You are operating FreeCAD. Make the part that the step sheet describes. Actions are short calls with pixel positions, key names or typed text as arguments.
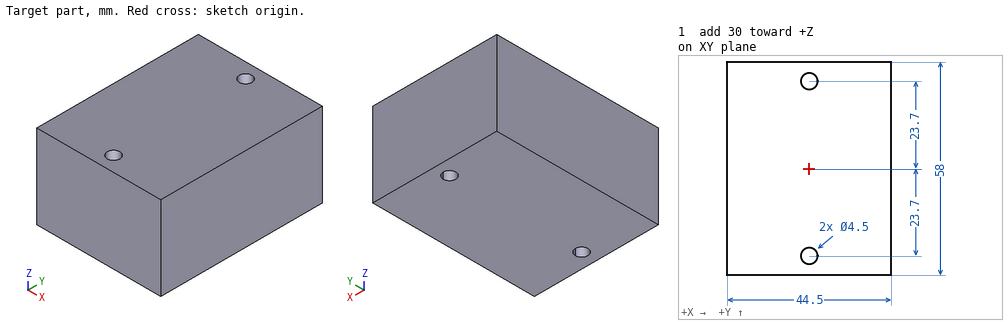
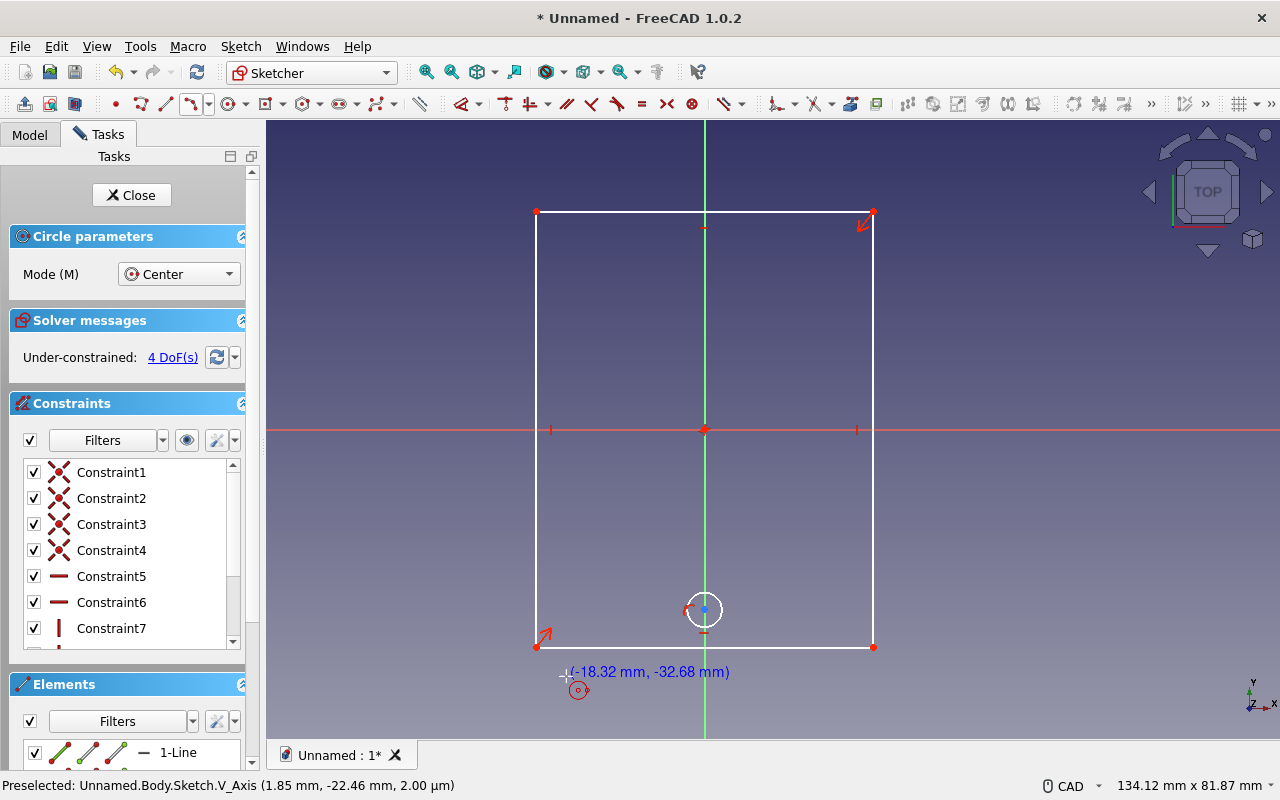
scroll(705, 251, up, 2)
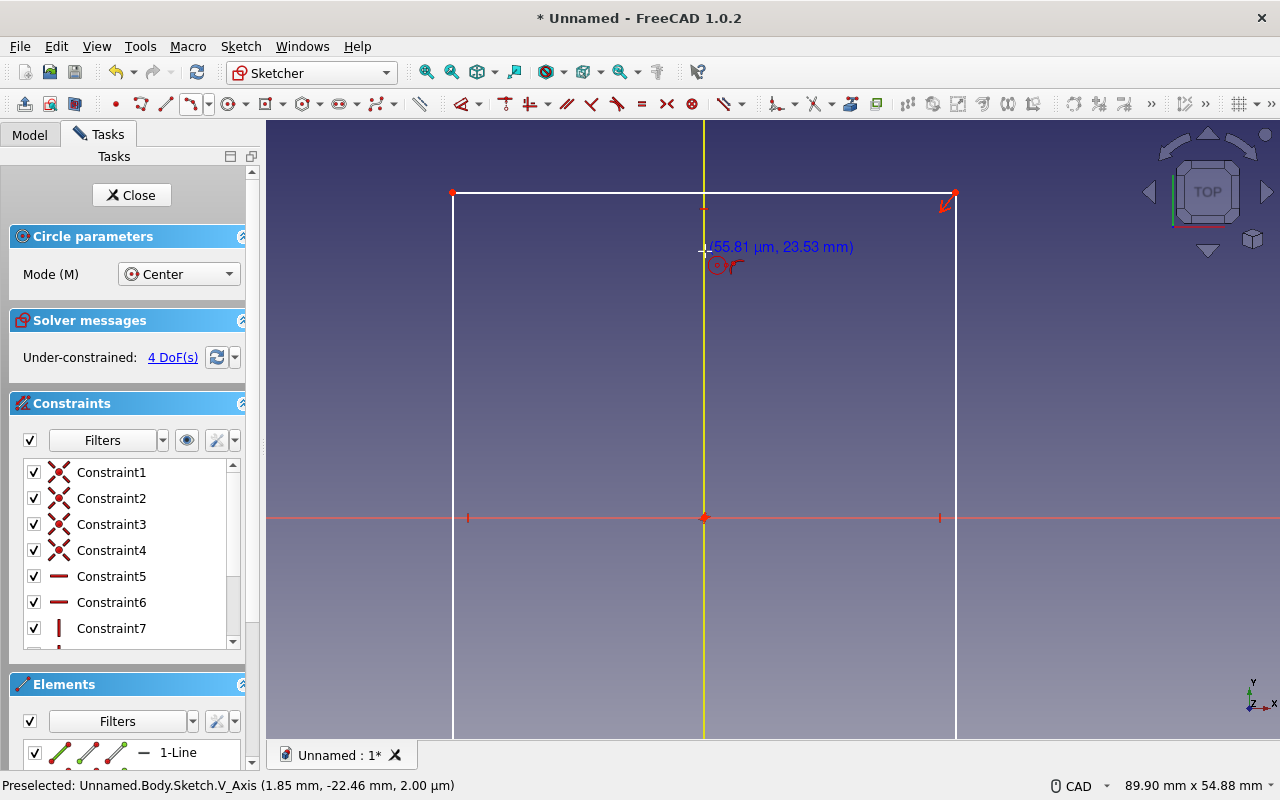
click(704, 251)
click(722, 233)
key(Escape)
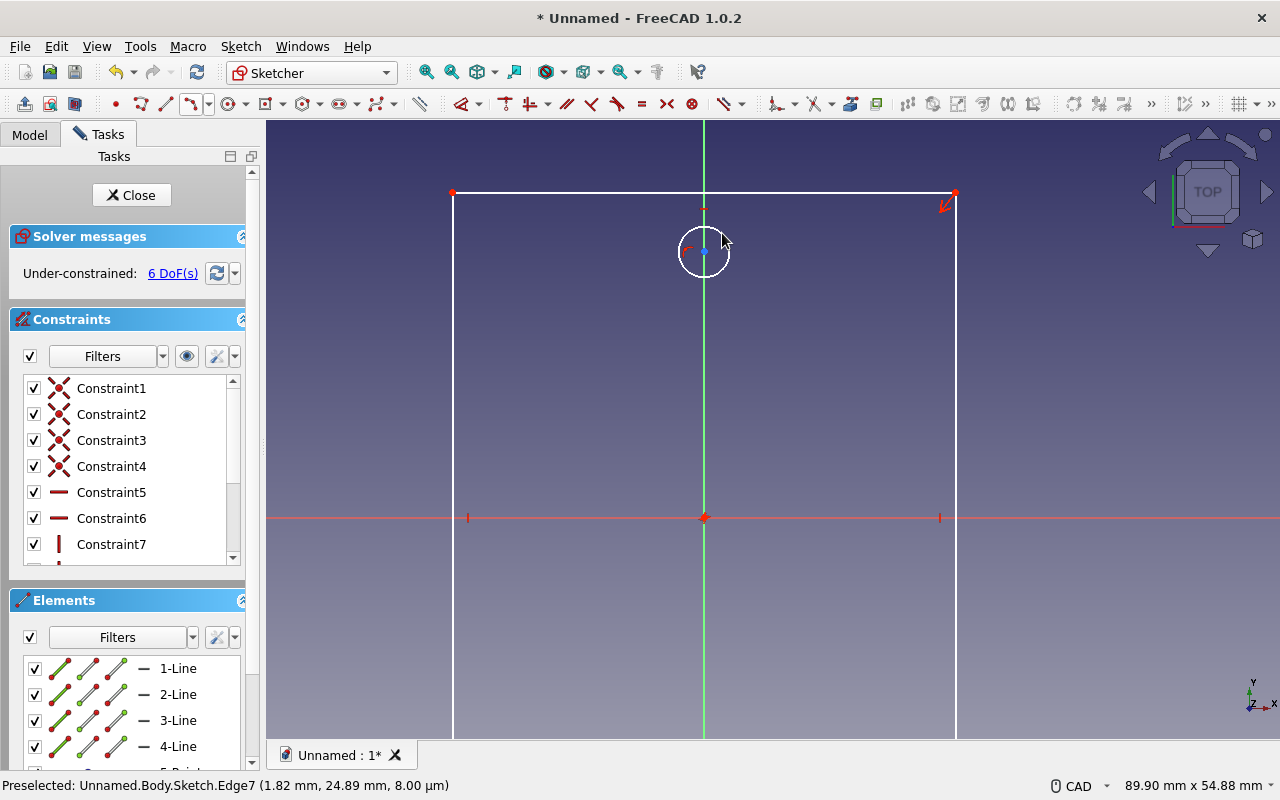
scroll(705, 250, down, 2)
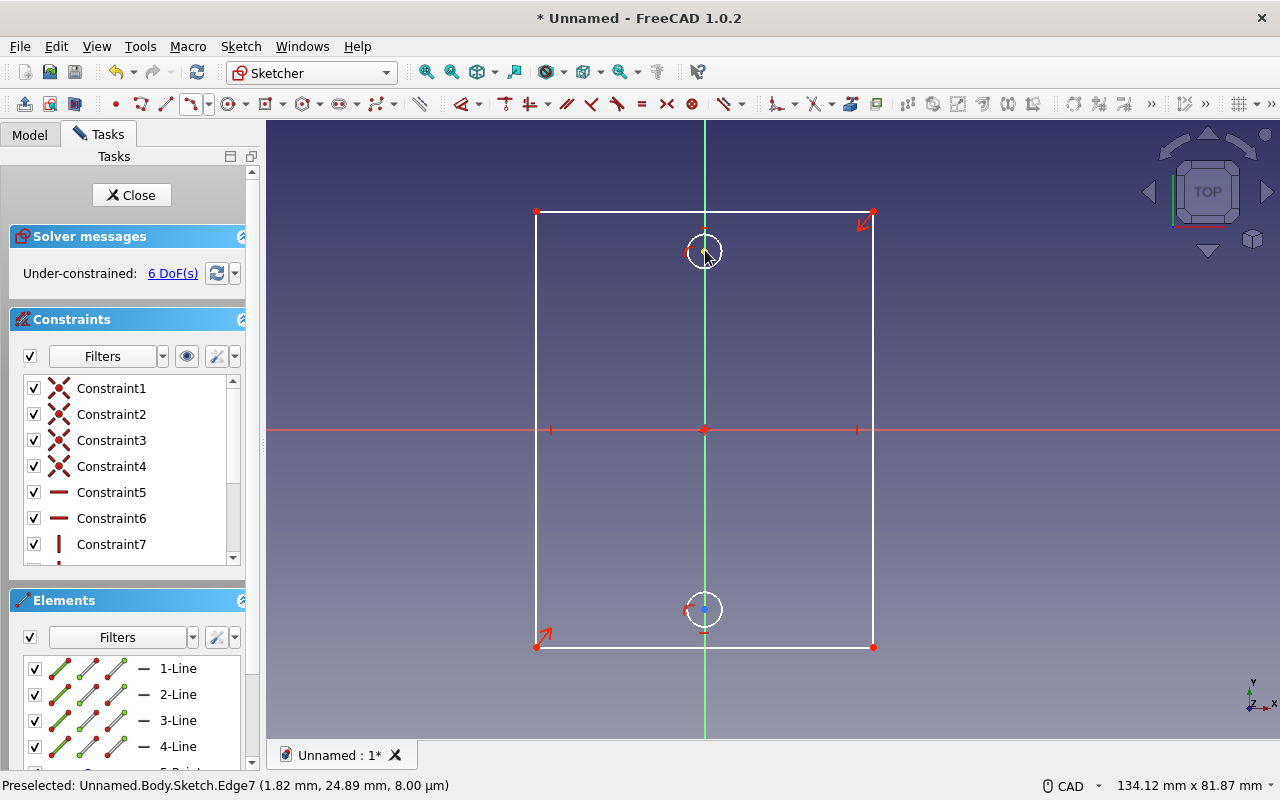
click(717, 597)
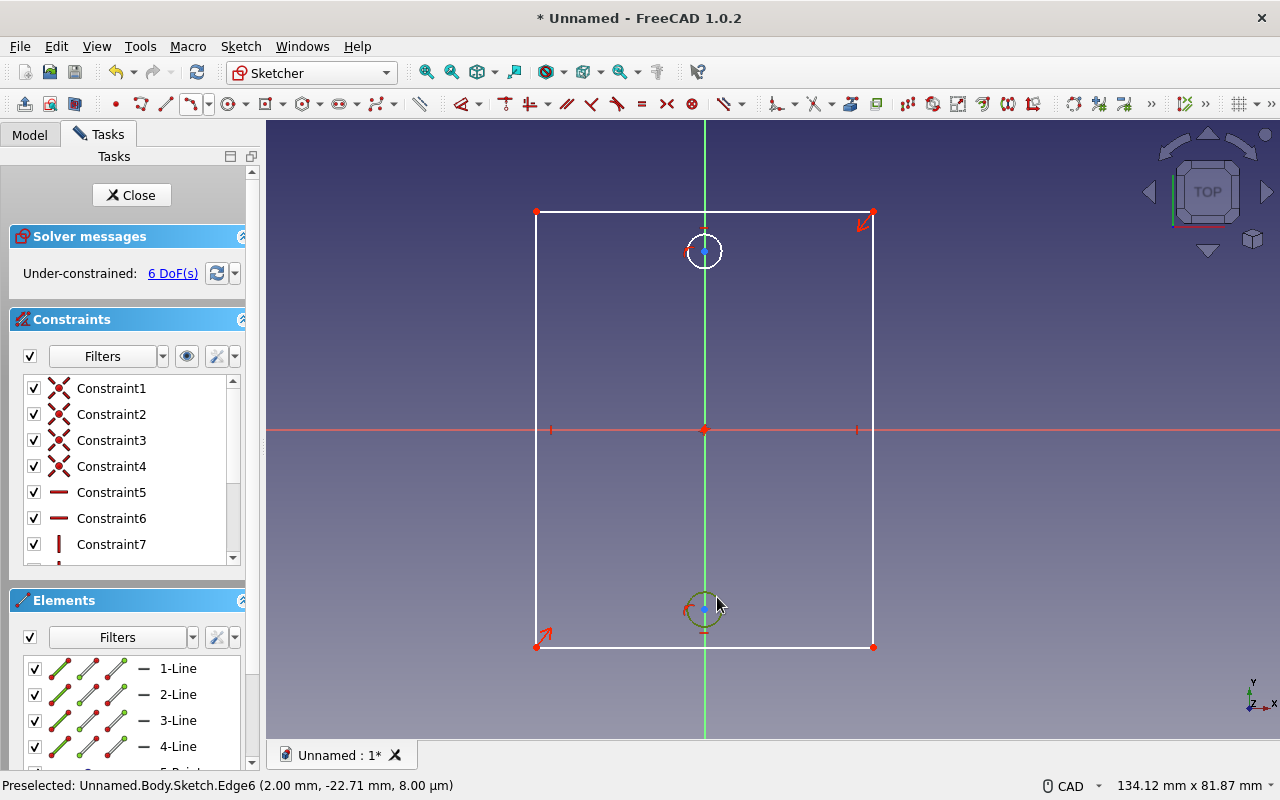
click(717, 239)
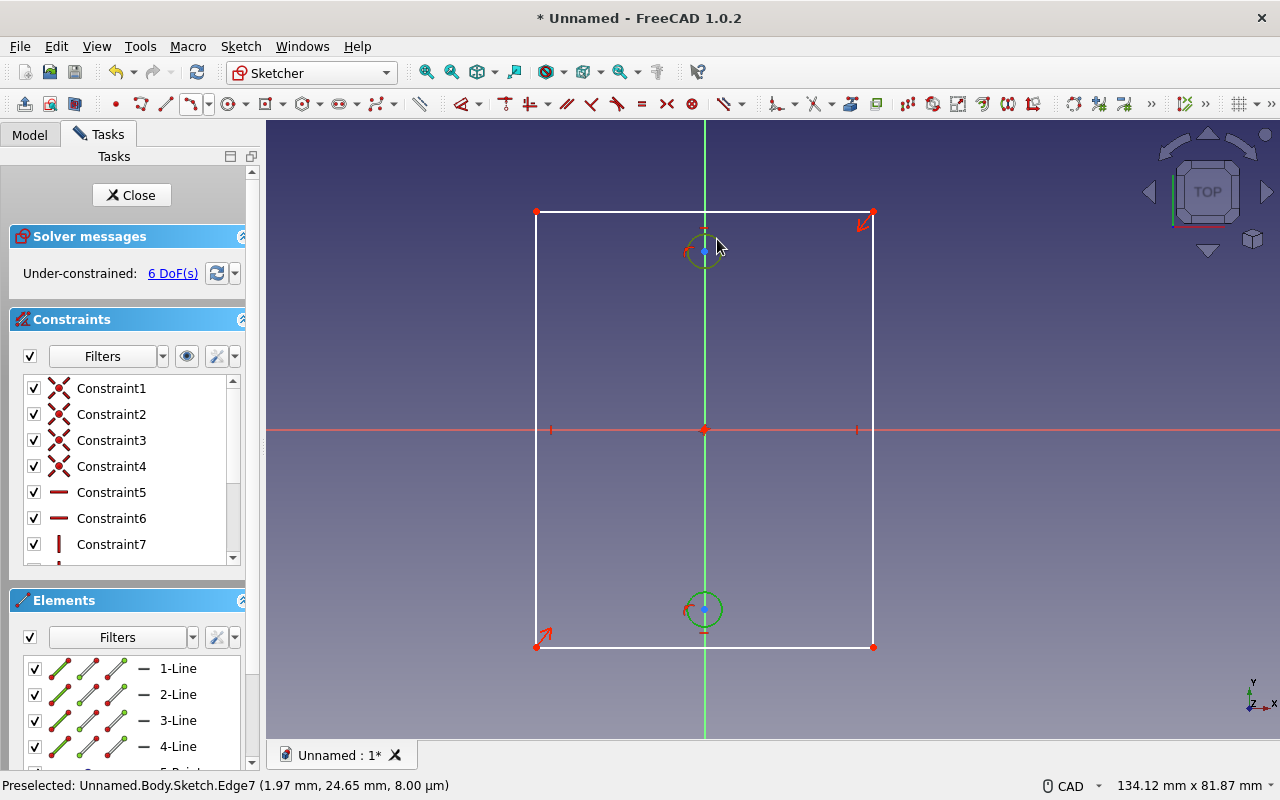
click(642, 104)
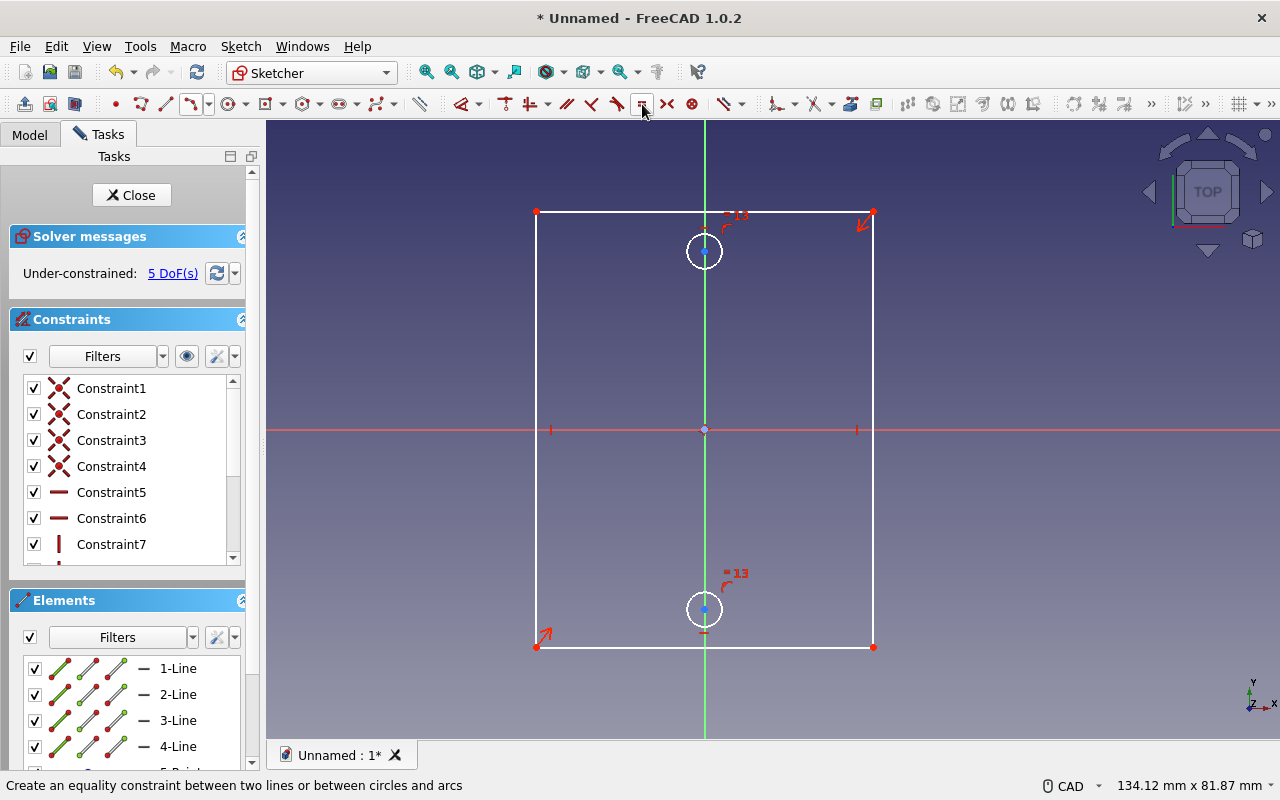
click(460, 104)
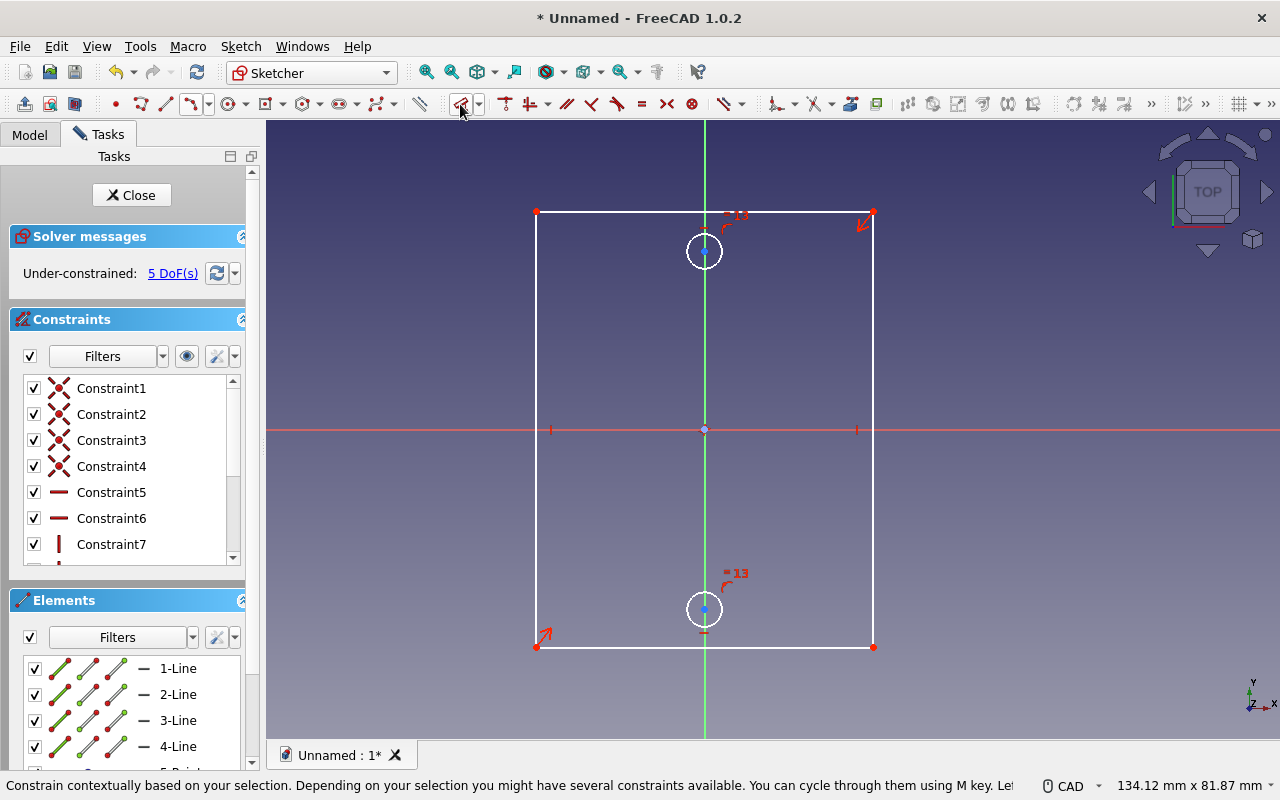
click(717, 597)
click(739, 574)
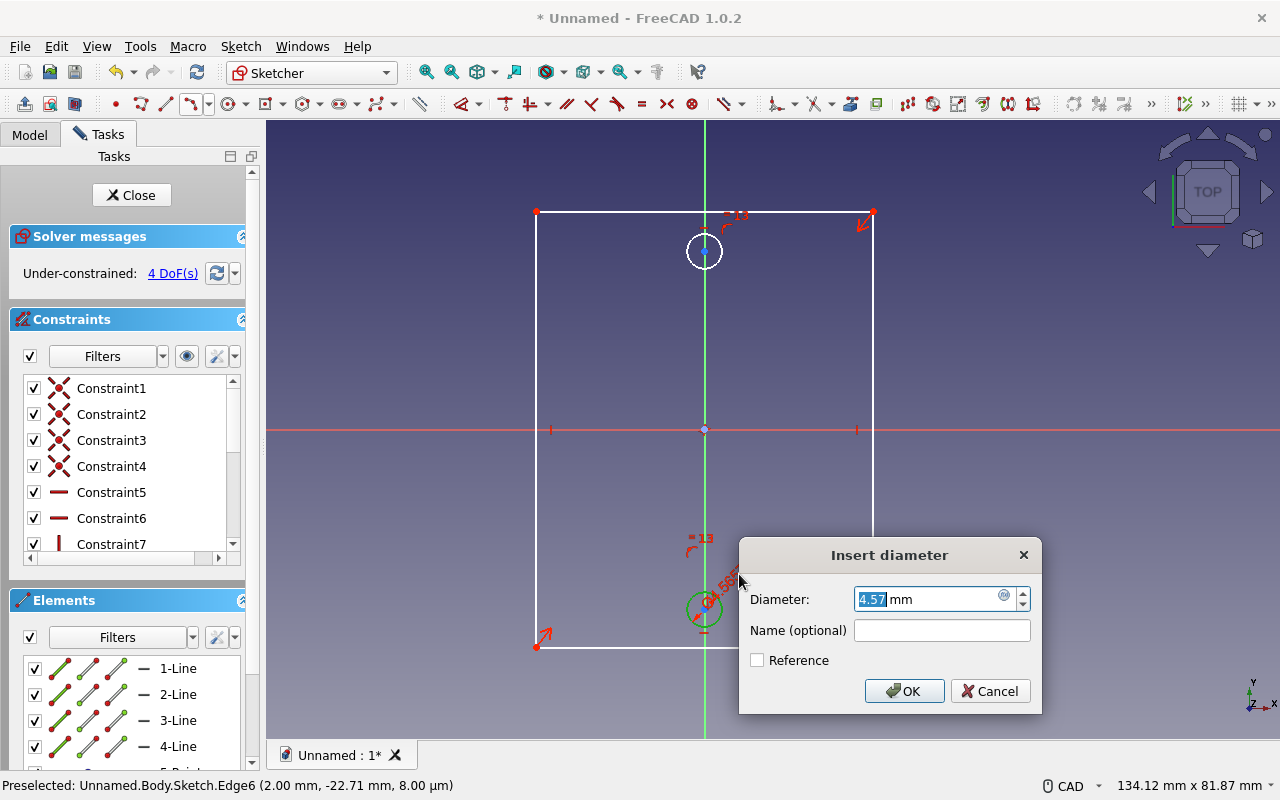
text(4.5)
key(Return)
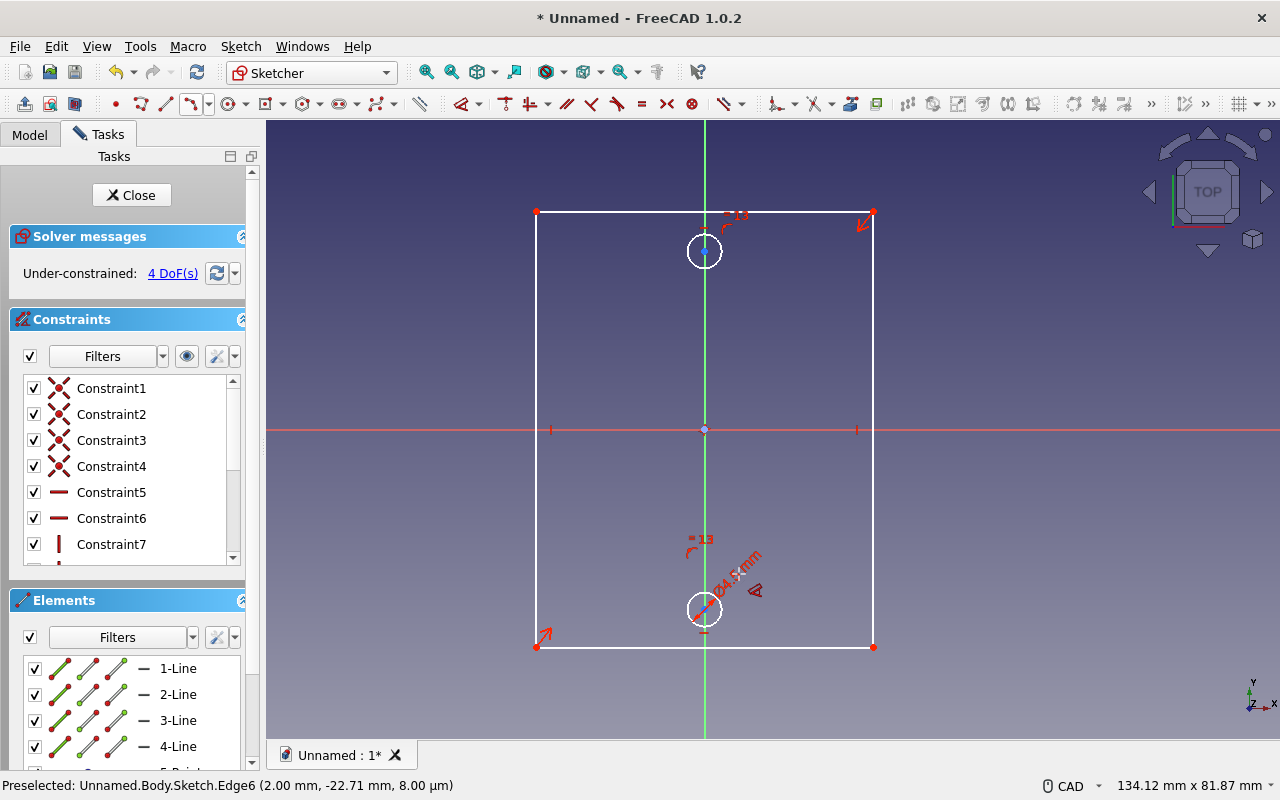
click(873, 517)
click(907, 329)